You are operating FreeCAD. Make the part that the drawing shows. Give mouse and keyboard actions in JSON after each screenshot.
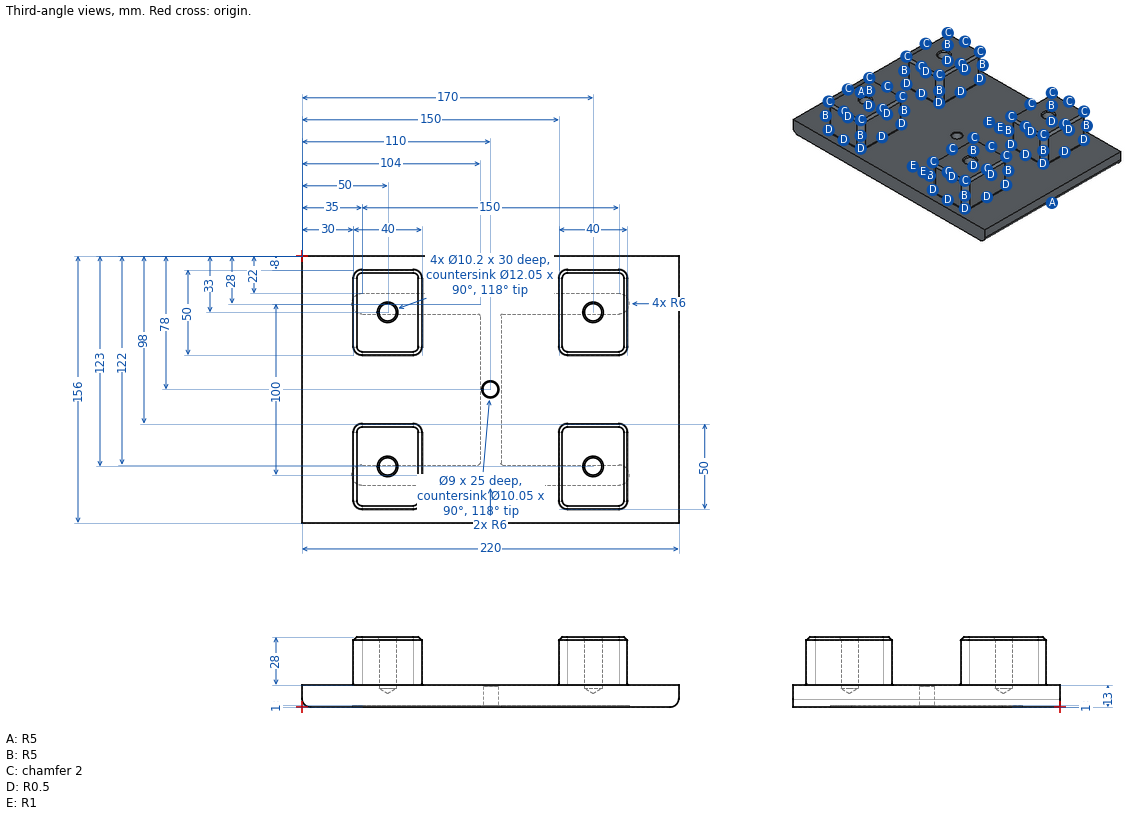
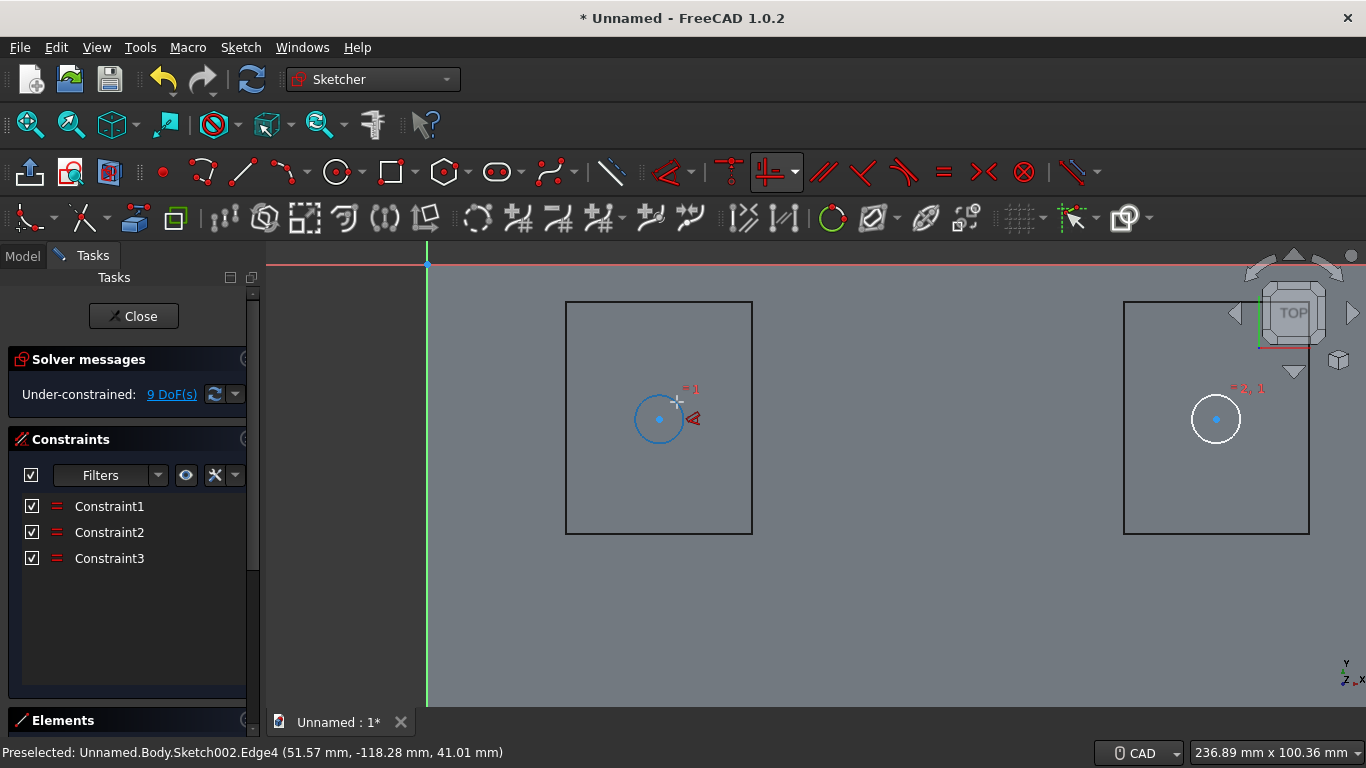
{"action": "left_click", "coordinate": [676, 402]}
{"action": "left_click", "coordinate": [698, 379]}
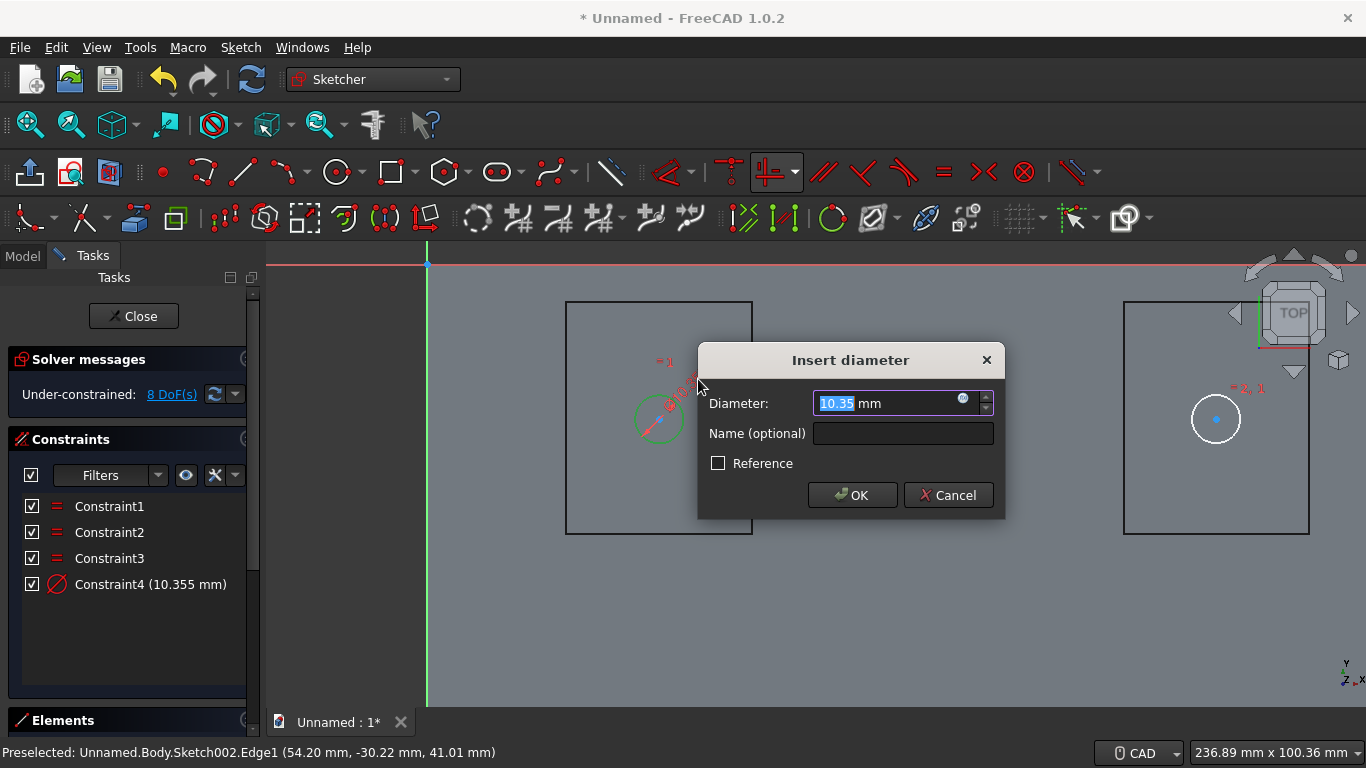
{"action": "type", "text": "10.2"}
{"action": "key", "text": "Return"}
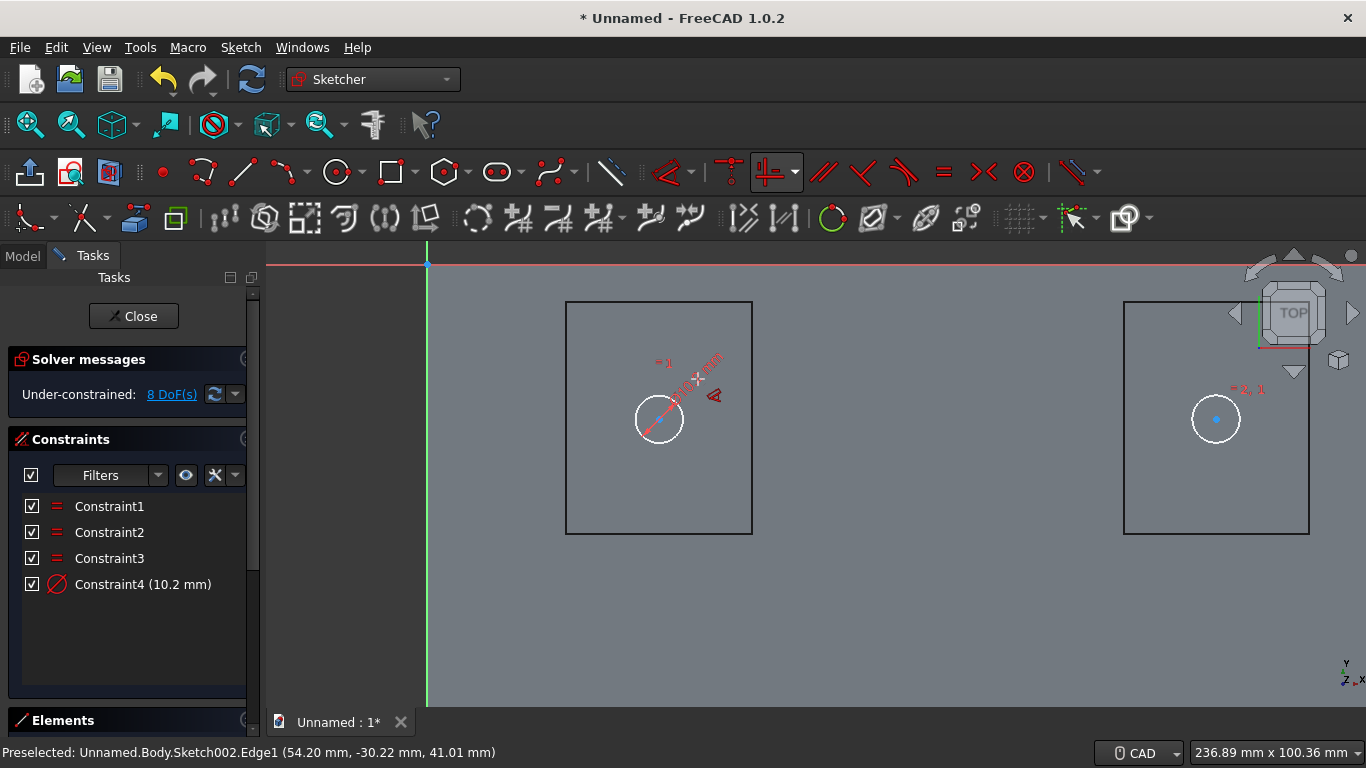
{"action": "left_click", "coordinate": [659, 419]}
{"action": "left_click", "coordinate": [543, 453]}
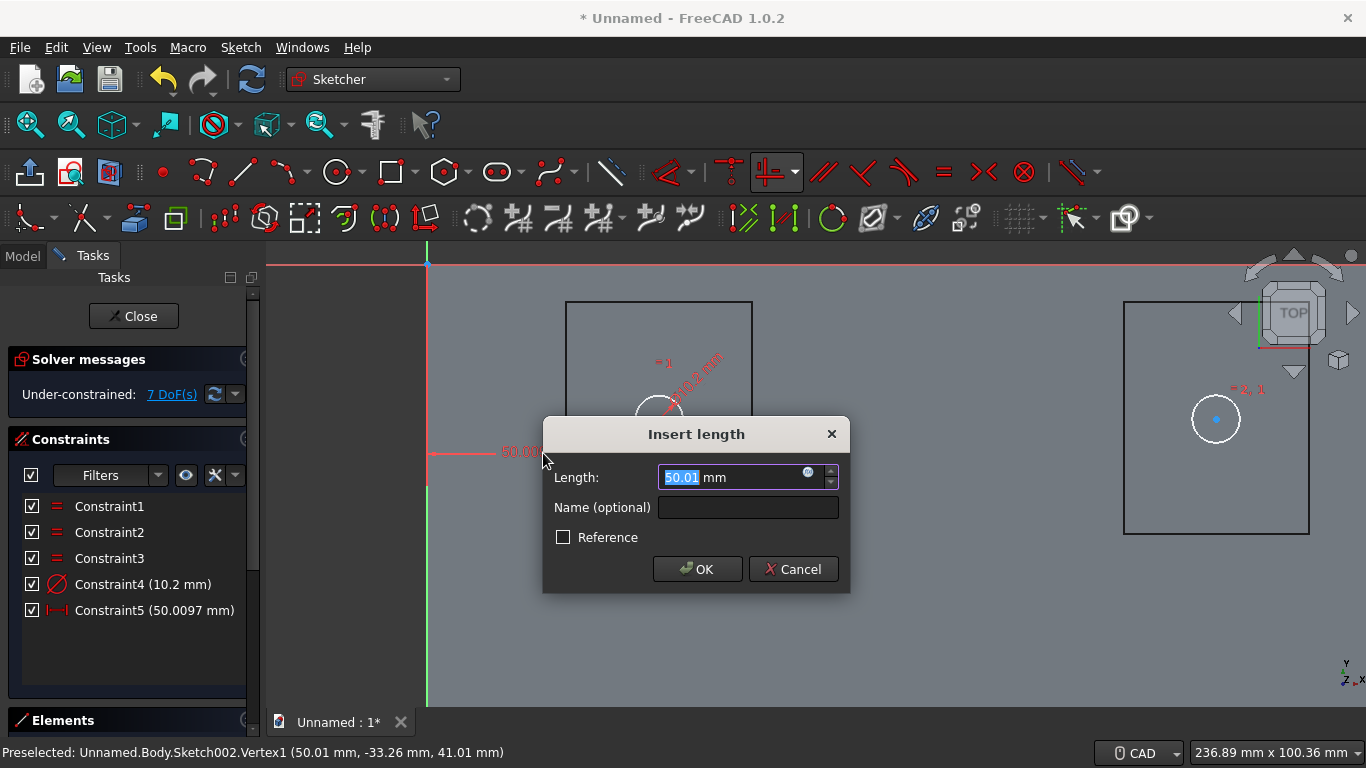
{"action": "type", "text": "50"}
{"action": "key", "text": "Return"}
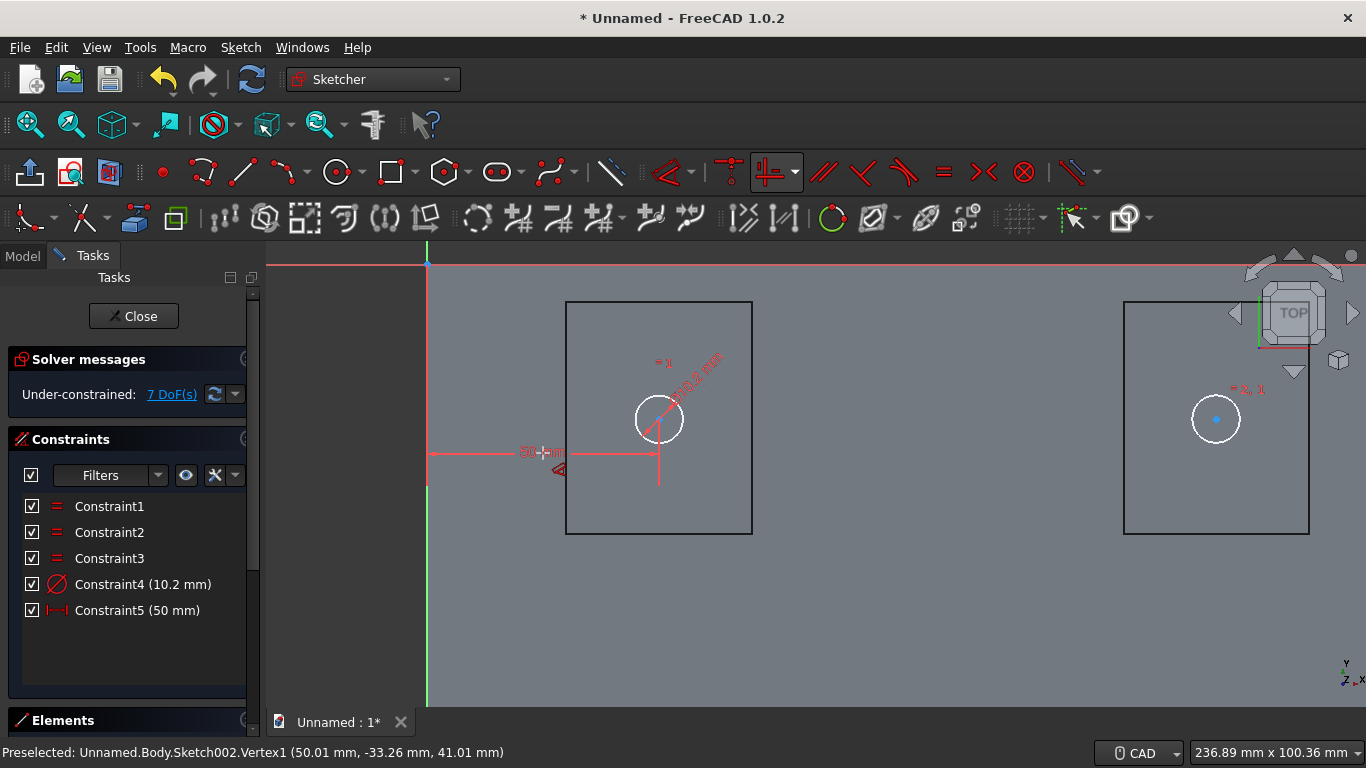
{"action": "left_click", "coordinate": [659, 419]}
{"action": "left_click", "coordinate": [393, 344]}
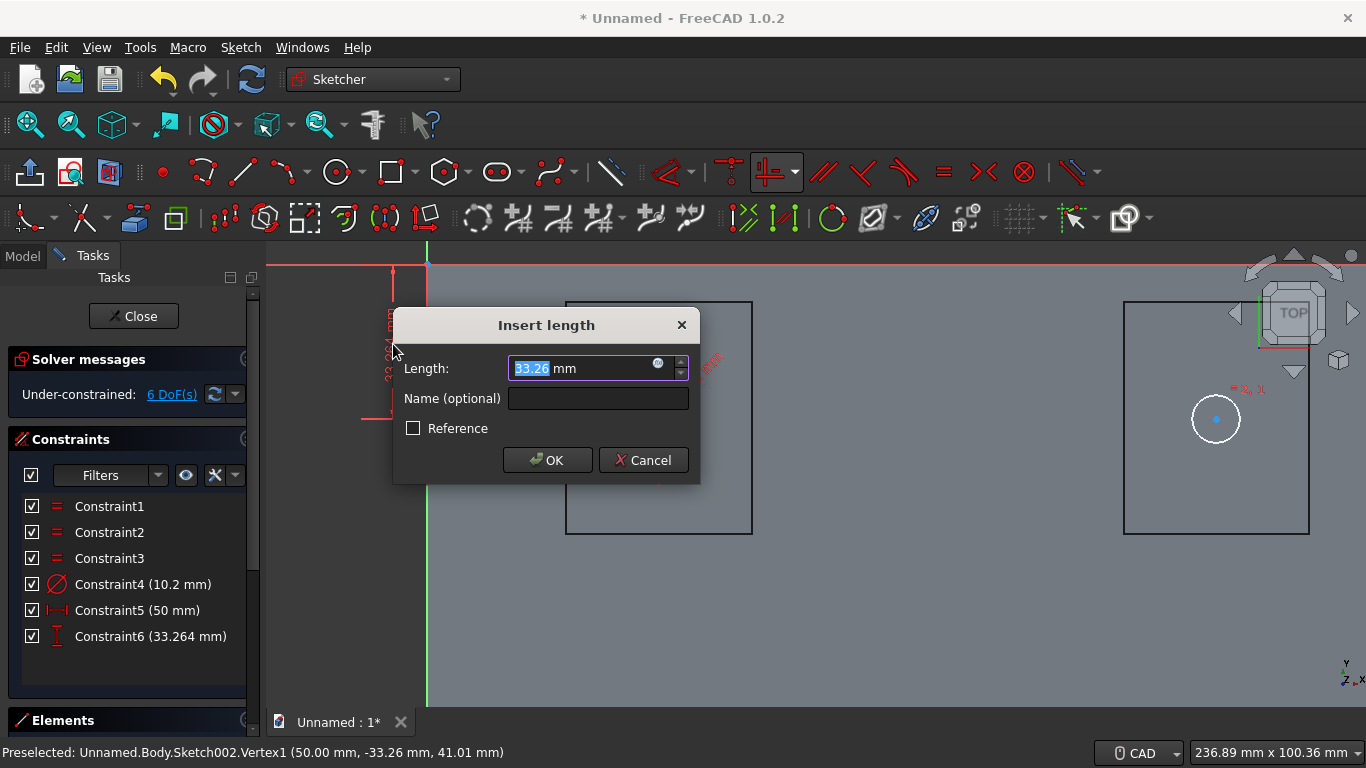
{"action": "type", "text": "33"}
{"action": "key", "text": "Return"}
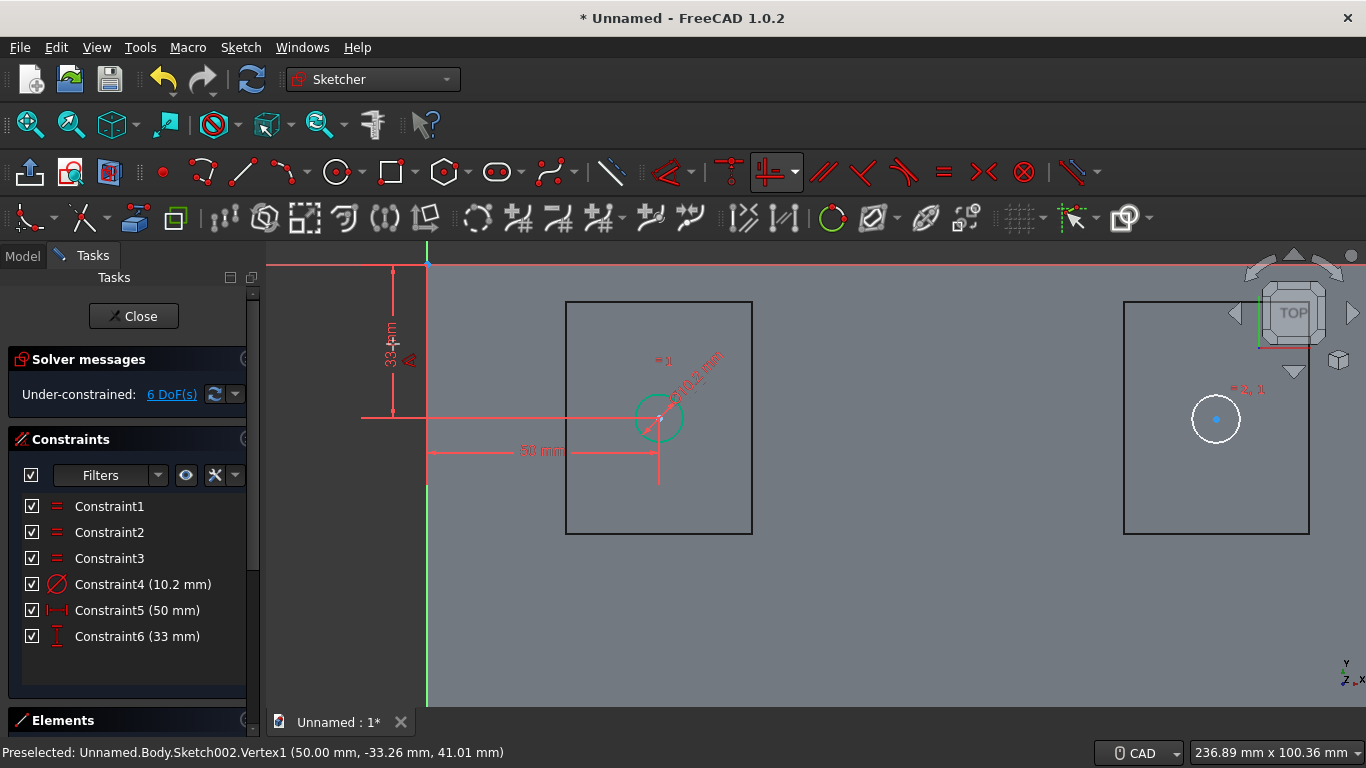
{"action": "scroll", "coordinate": [677, 402], "scroll_direction": "down", "scroll_amount": 4}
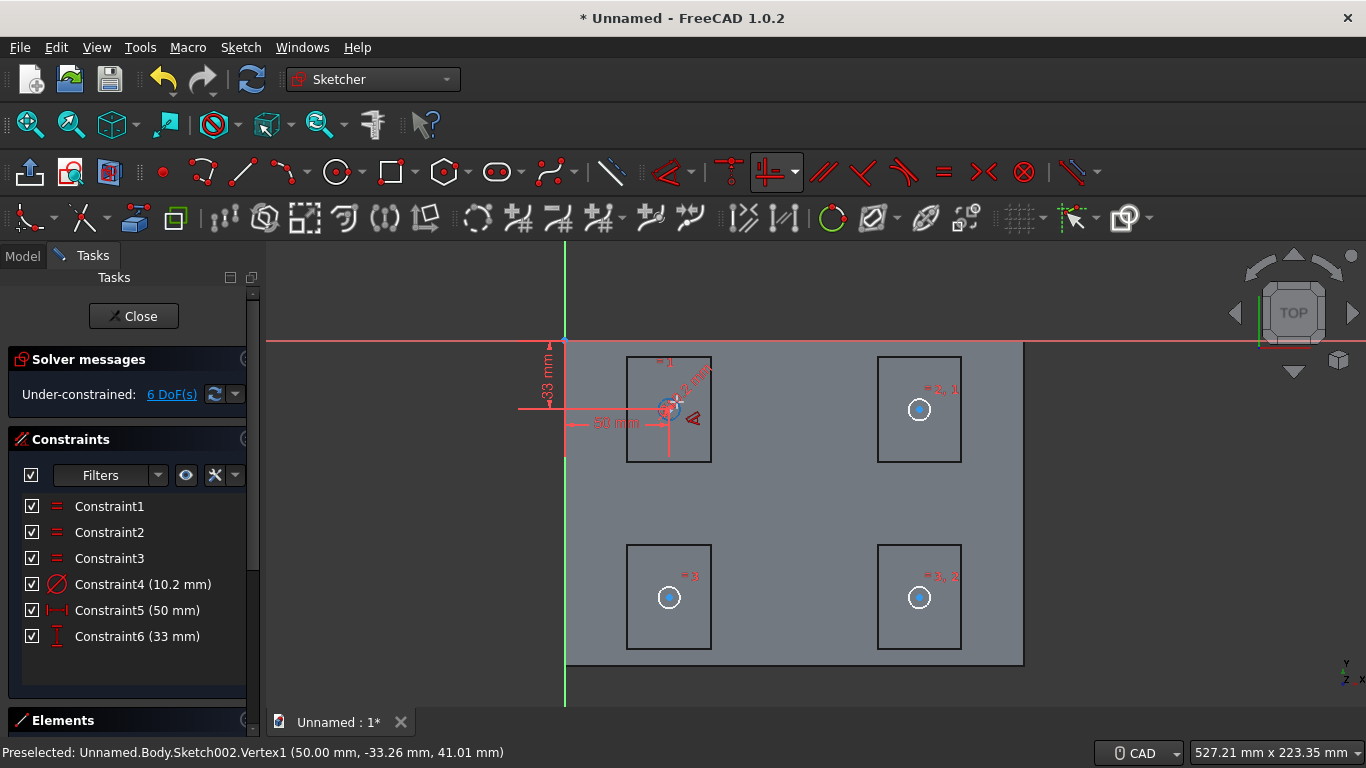
{"action": "left_click", "coordinate": [919, 410]}
{"action": "left_click", "coordinate": [531, 399]}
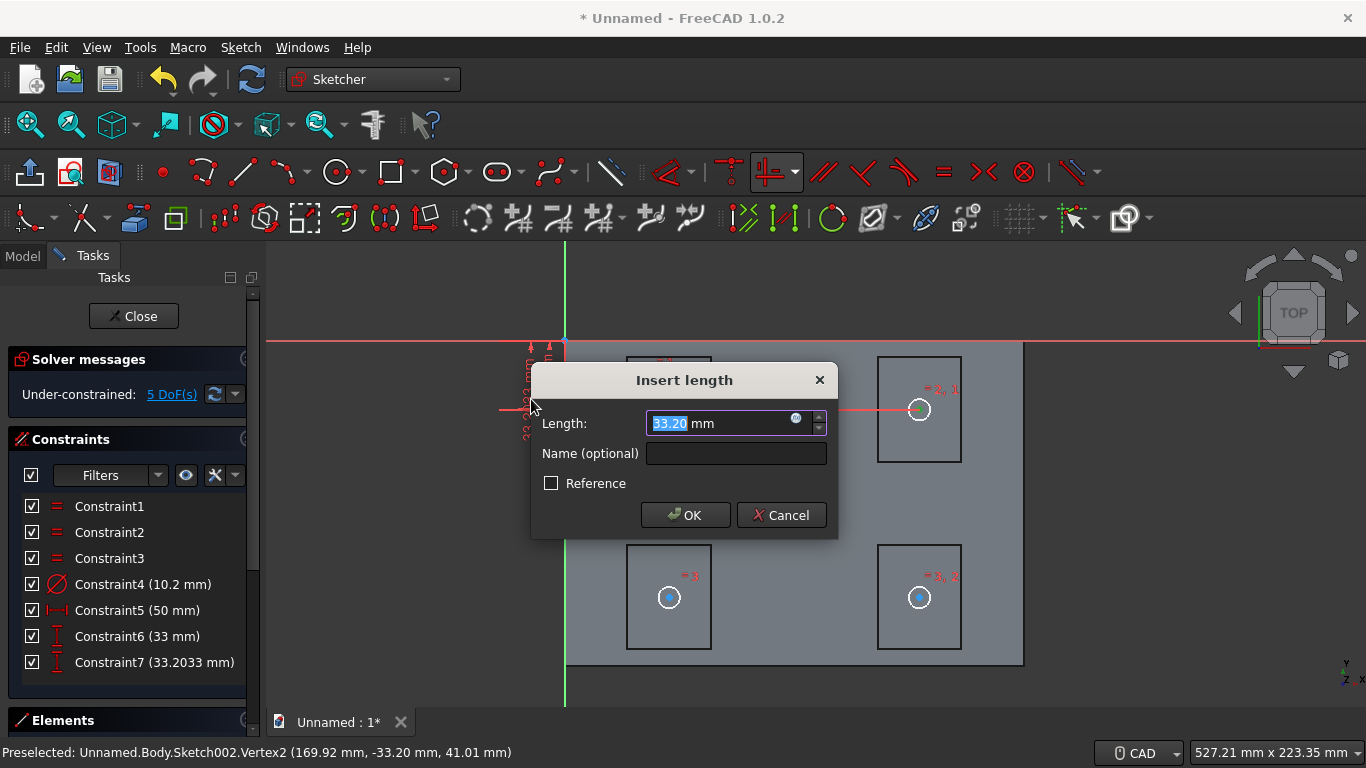
{"action": "type", "text": "33"}
{"action": "key", "text": "Return"}